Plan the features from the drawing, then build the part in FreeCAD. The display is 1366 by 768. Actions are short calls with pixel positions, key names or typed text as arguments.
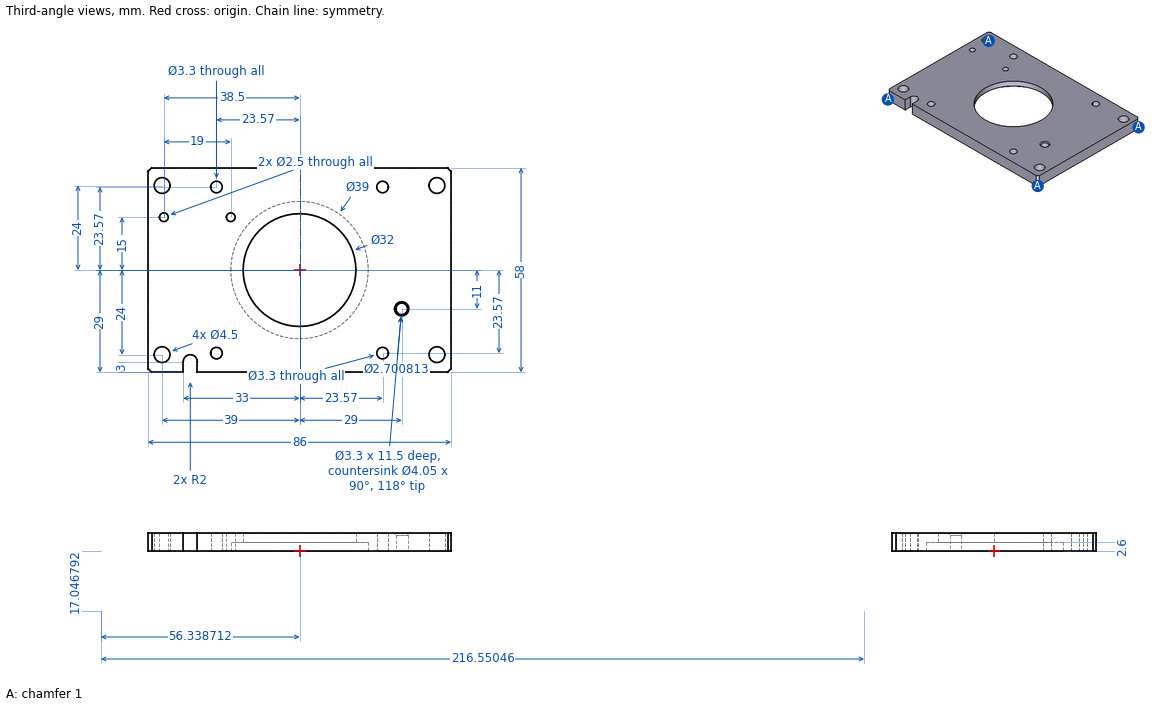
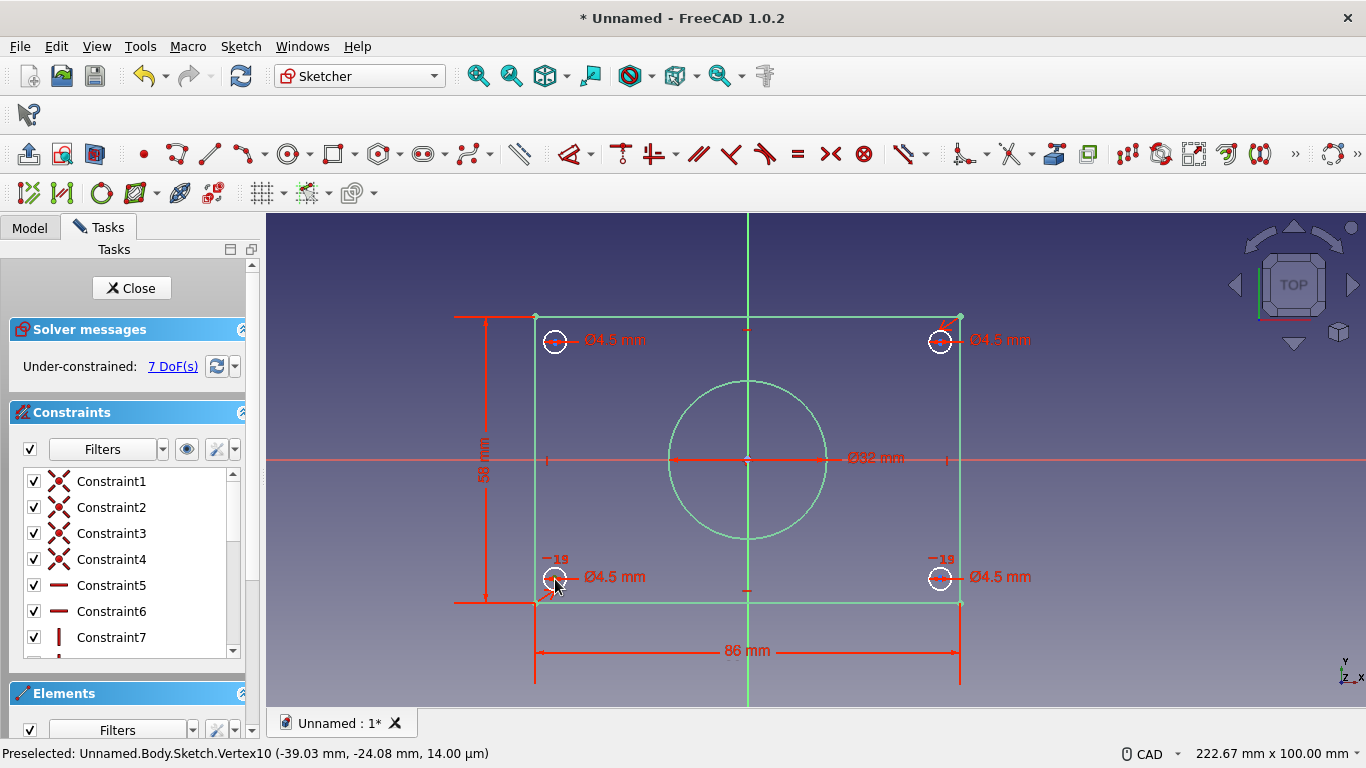
click(555, 342)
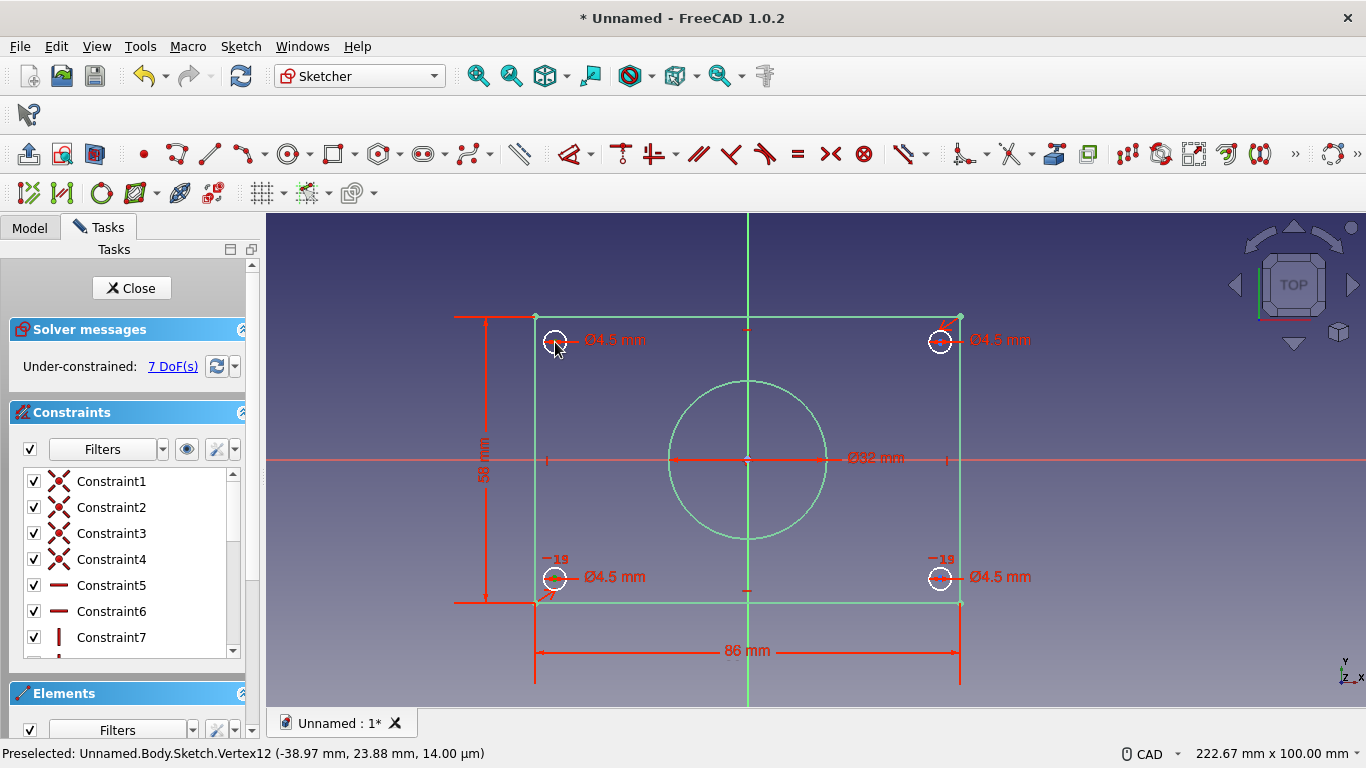
key(v)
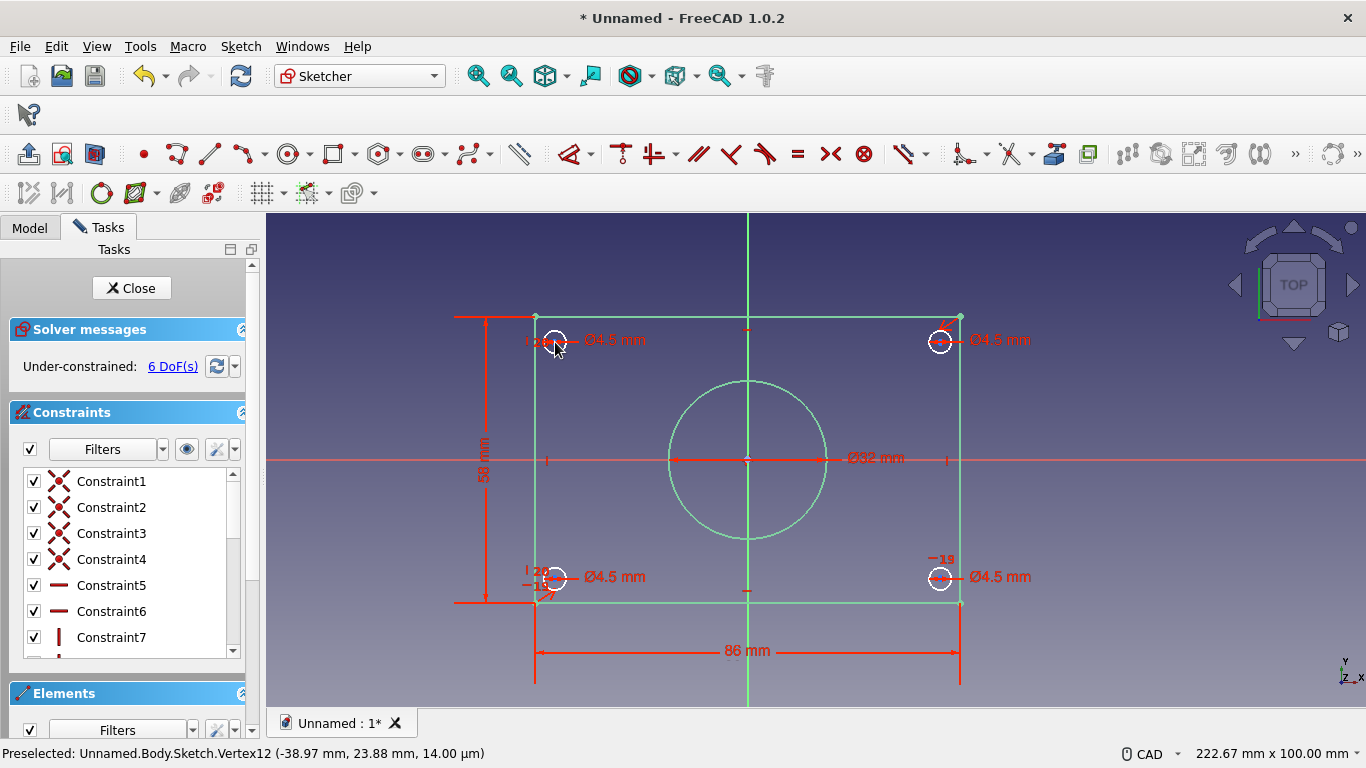
click(940, 579)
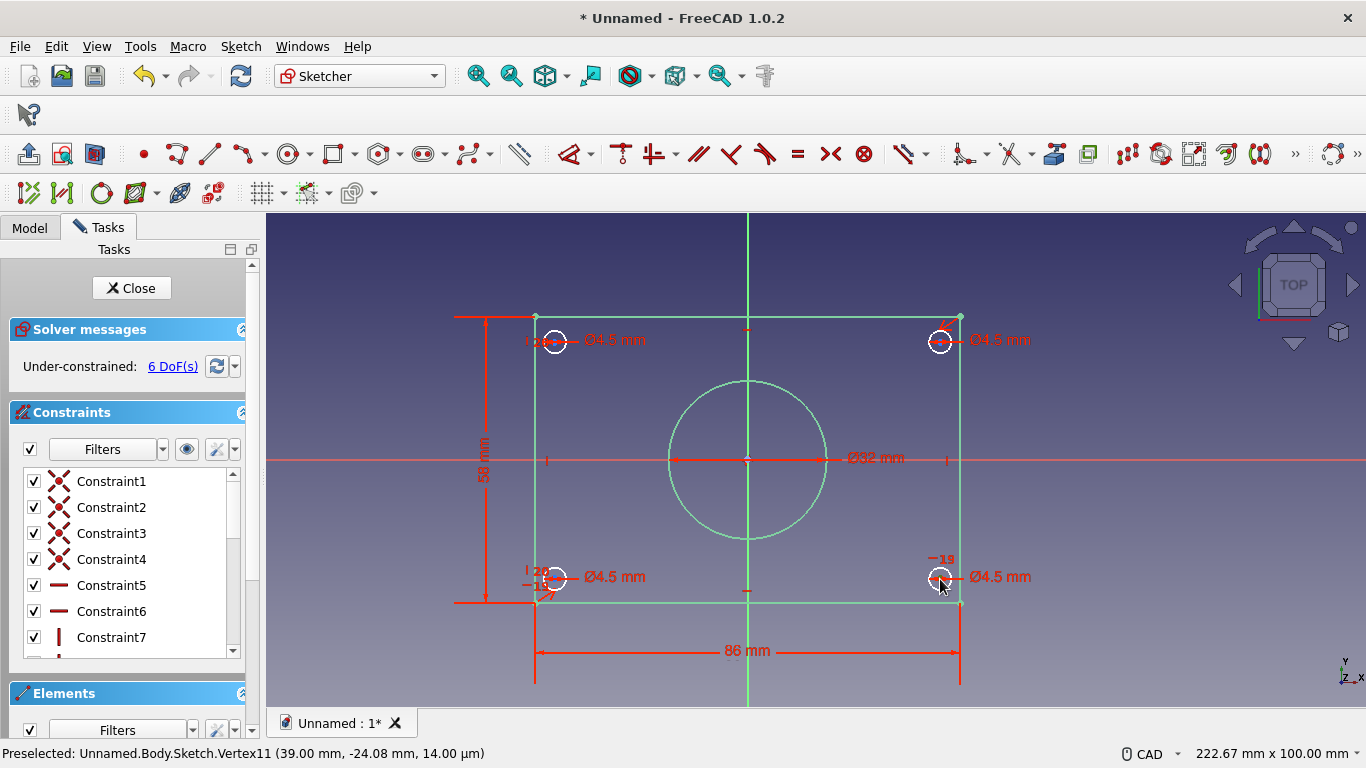
click(940, 342)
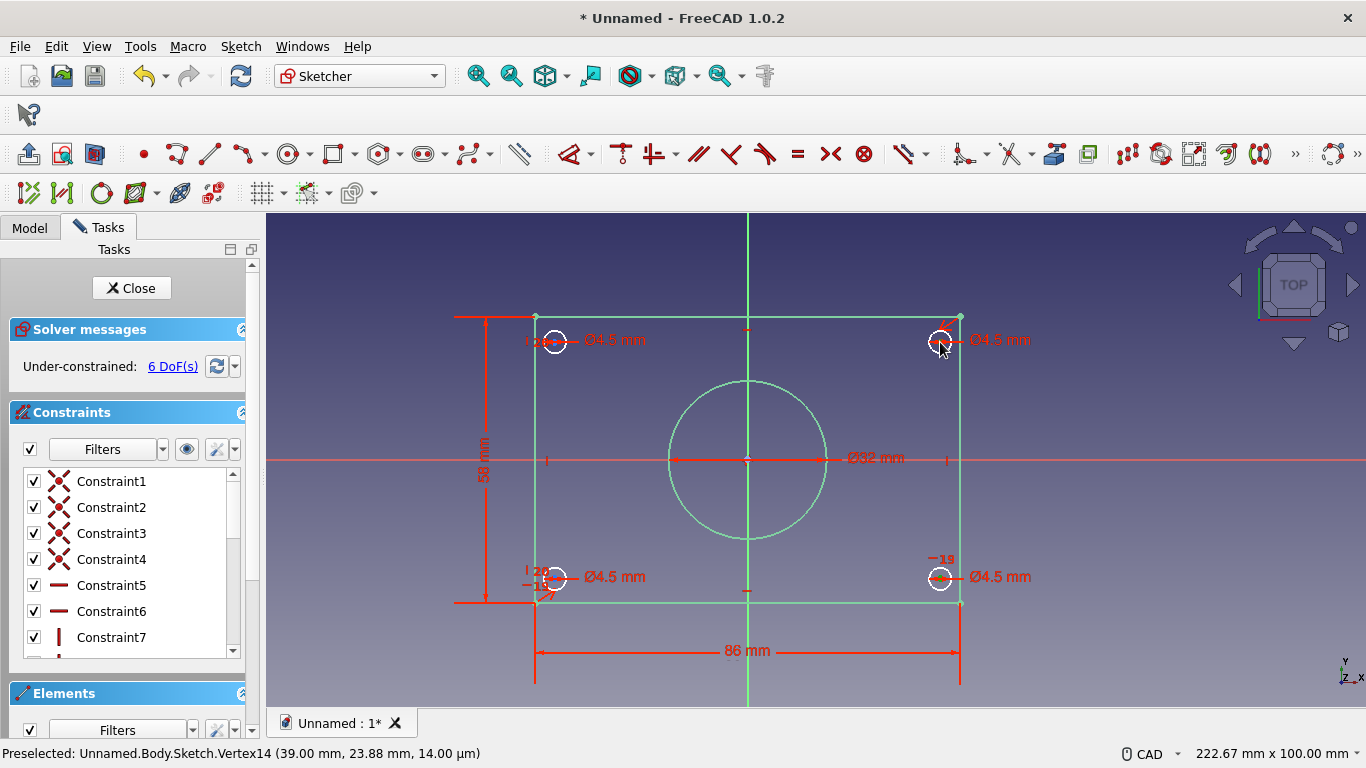
key(v)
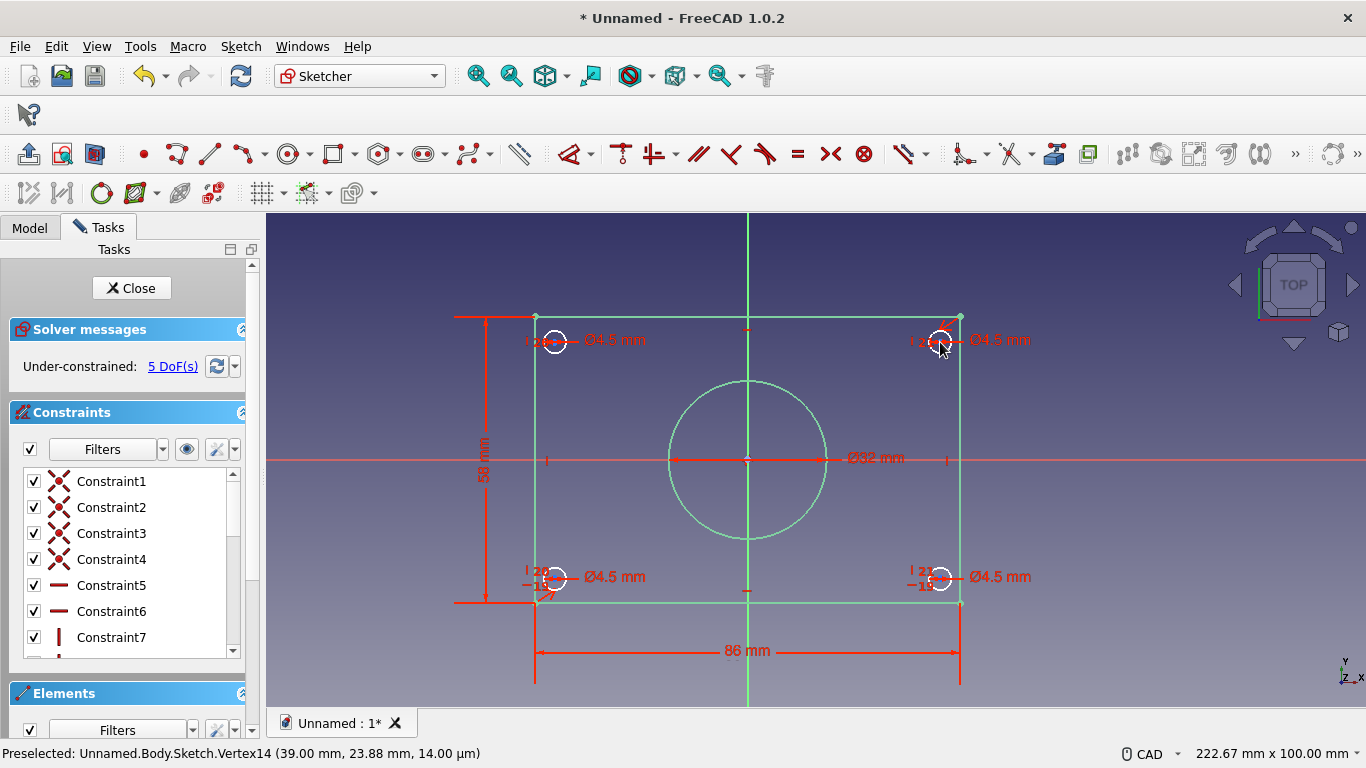
click(555, 342)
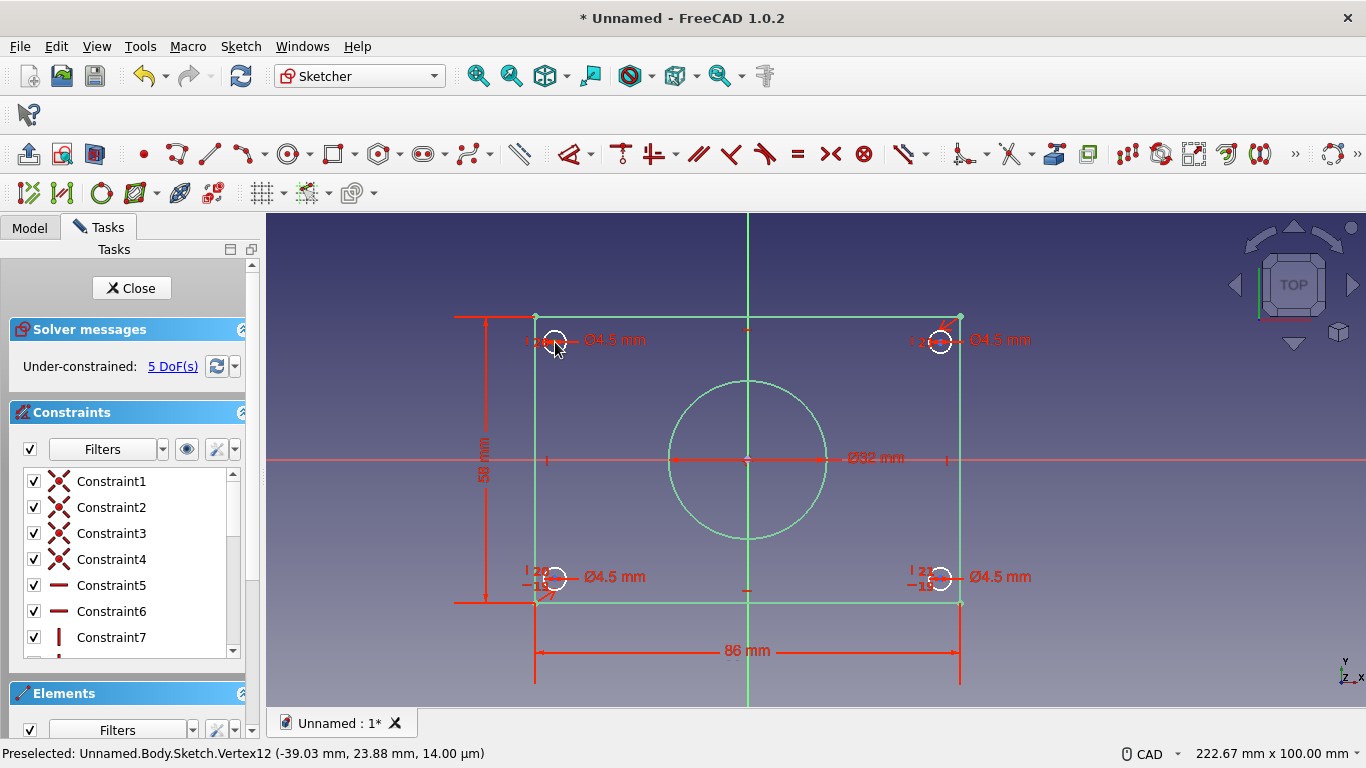
click(940, 342)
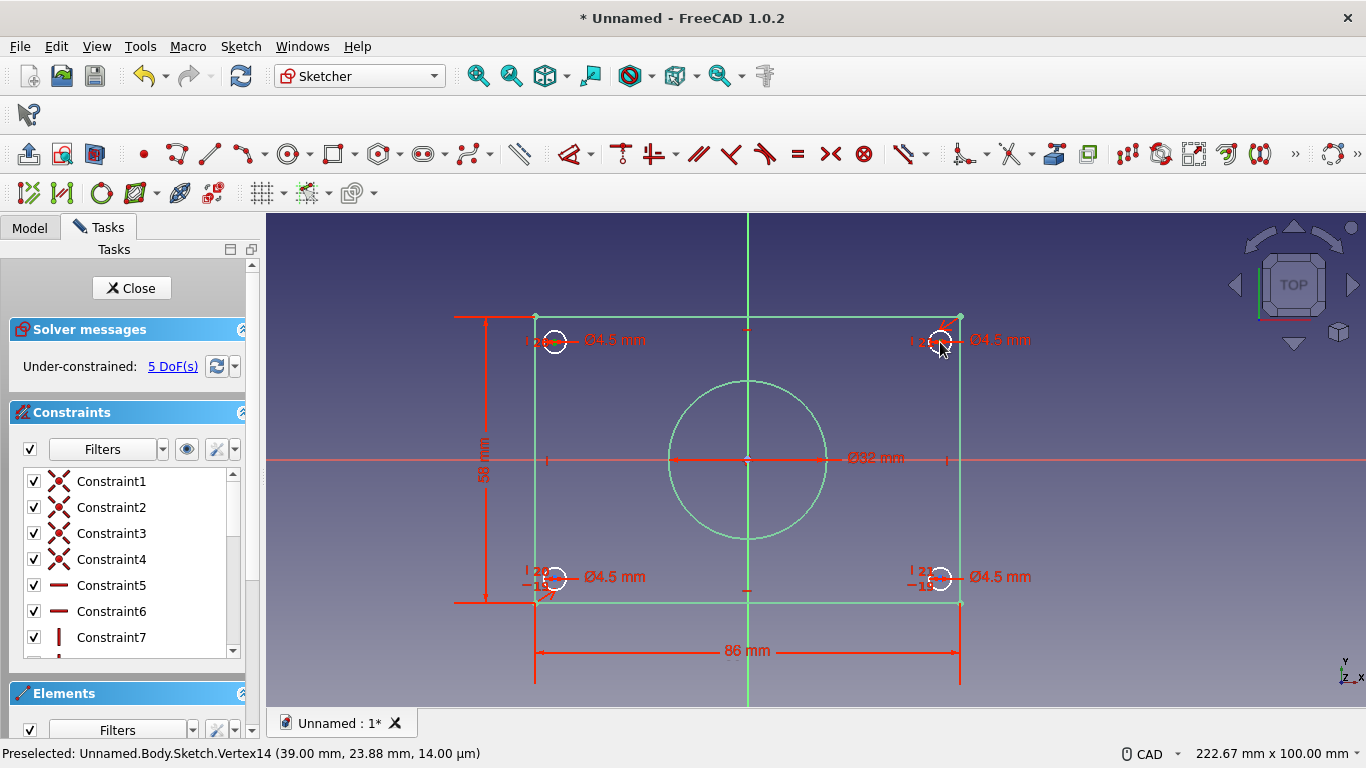
click(748, 491)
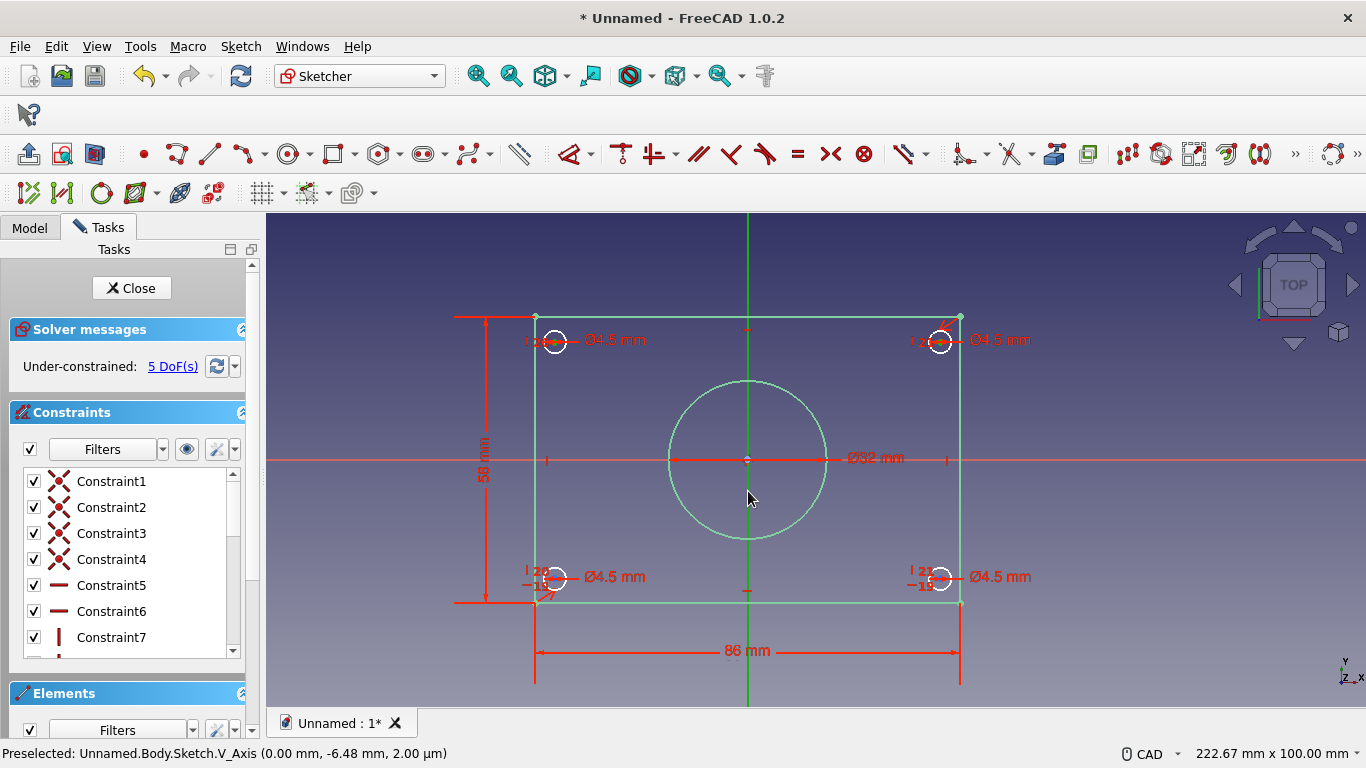
click(831, 154)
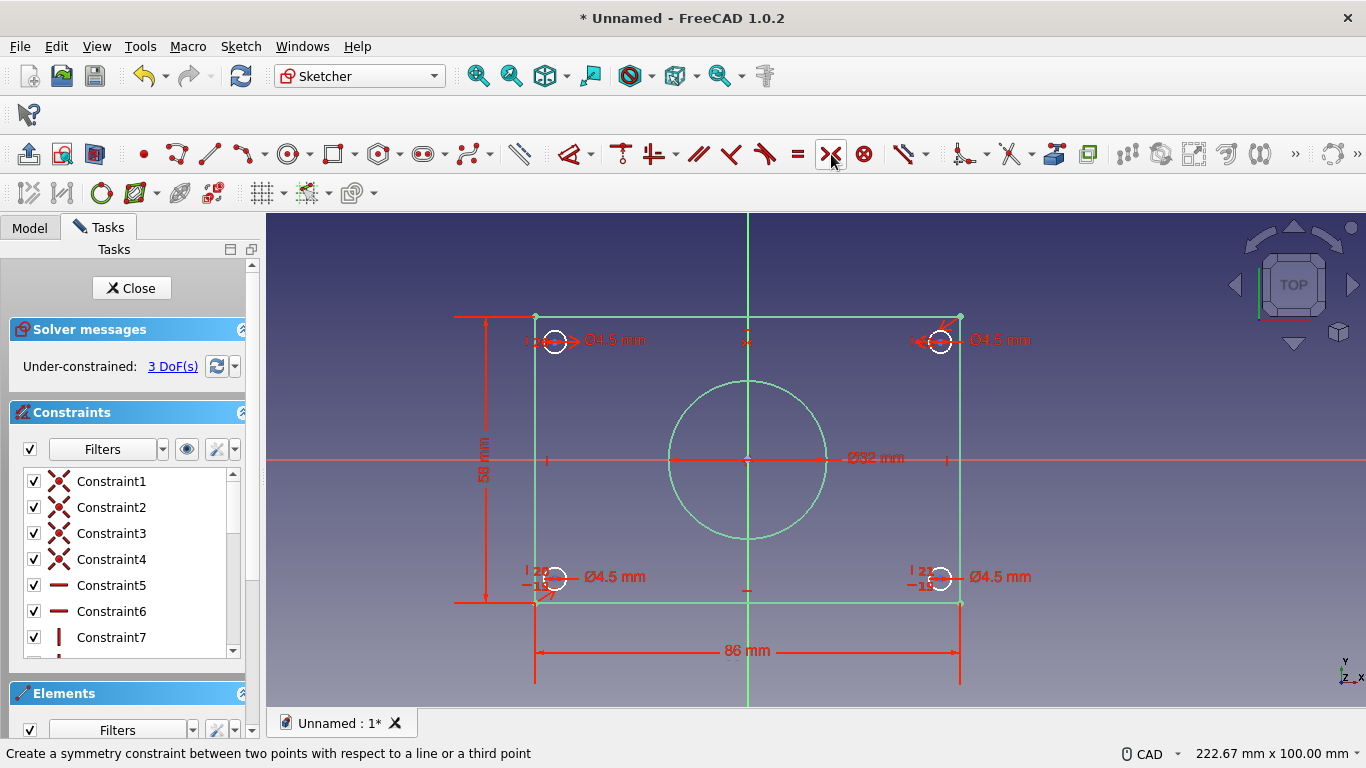
key(d)